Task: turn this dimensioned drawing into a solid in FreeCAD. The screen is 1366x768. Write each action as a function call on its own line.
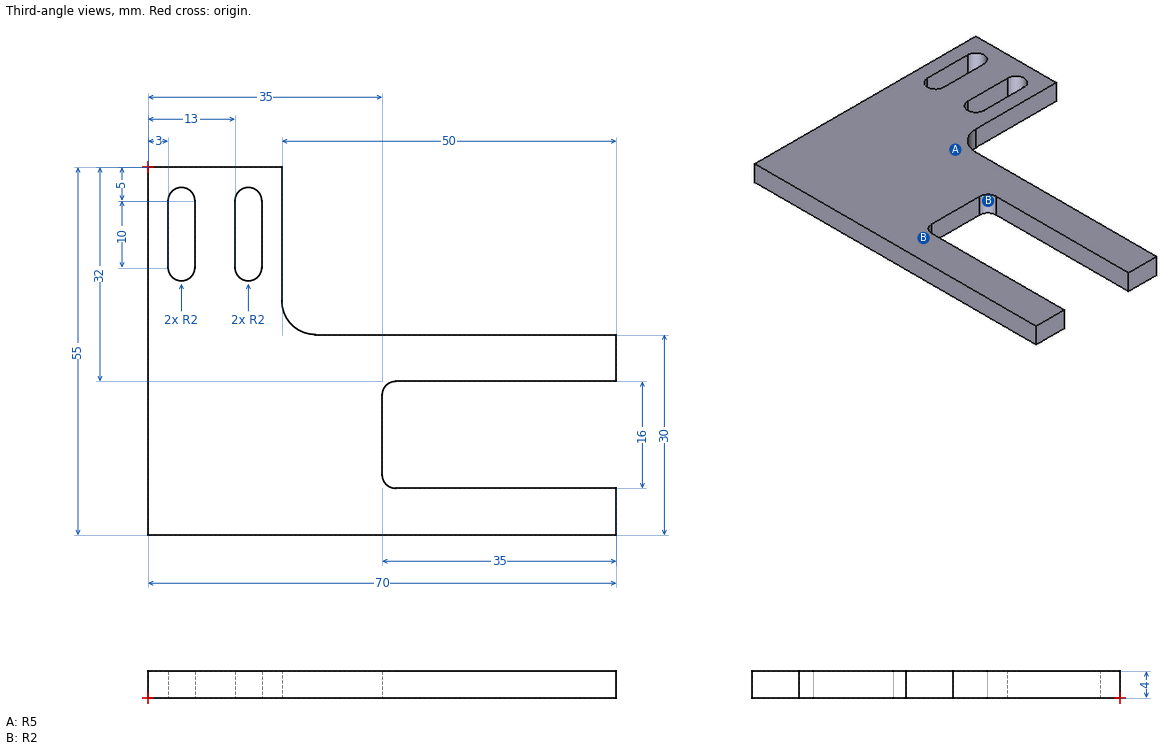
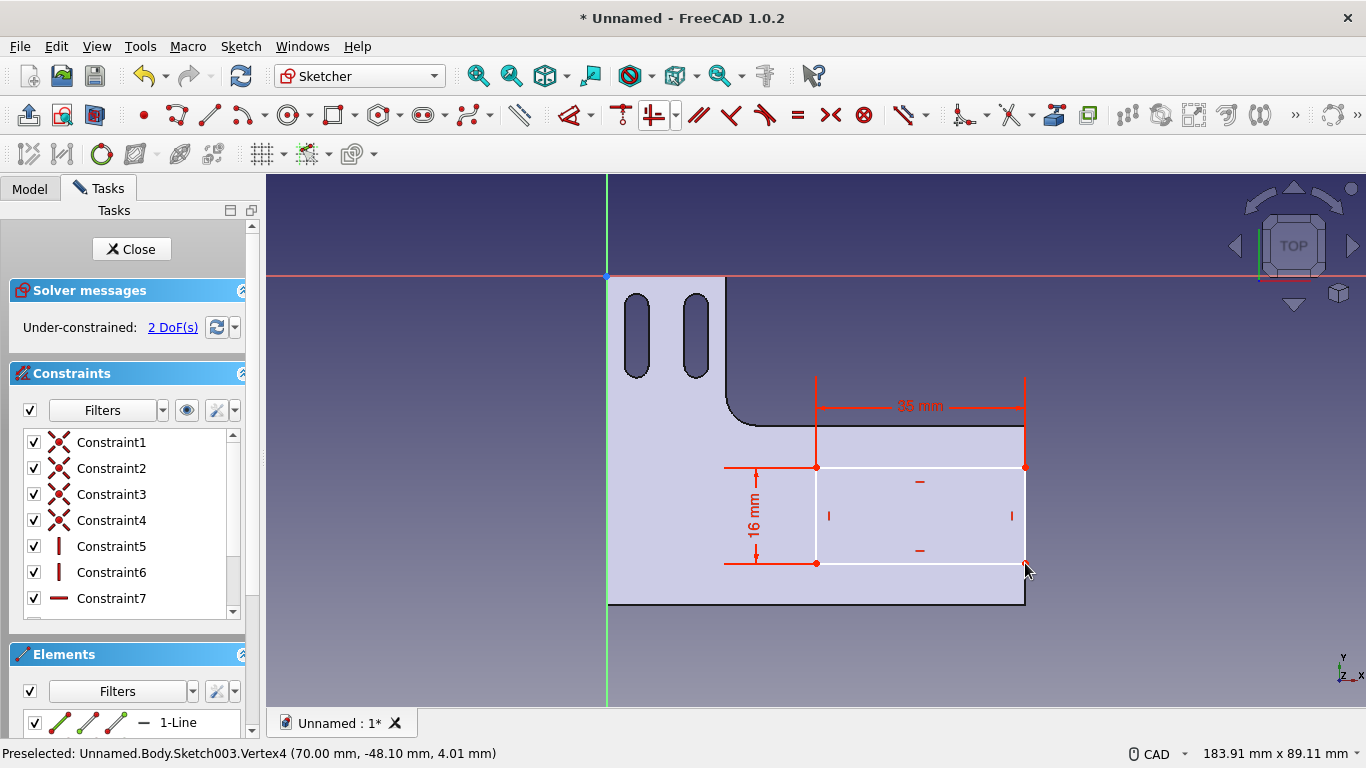
click(568, 116)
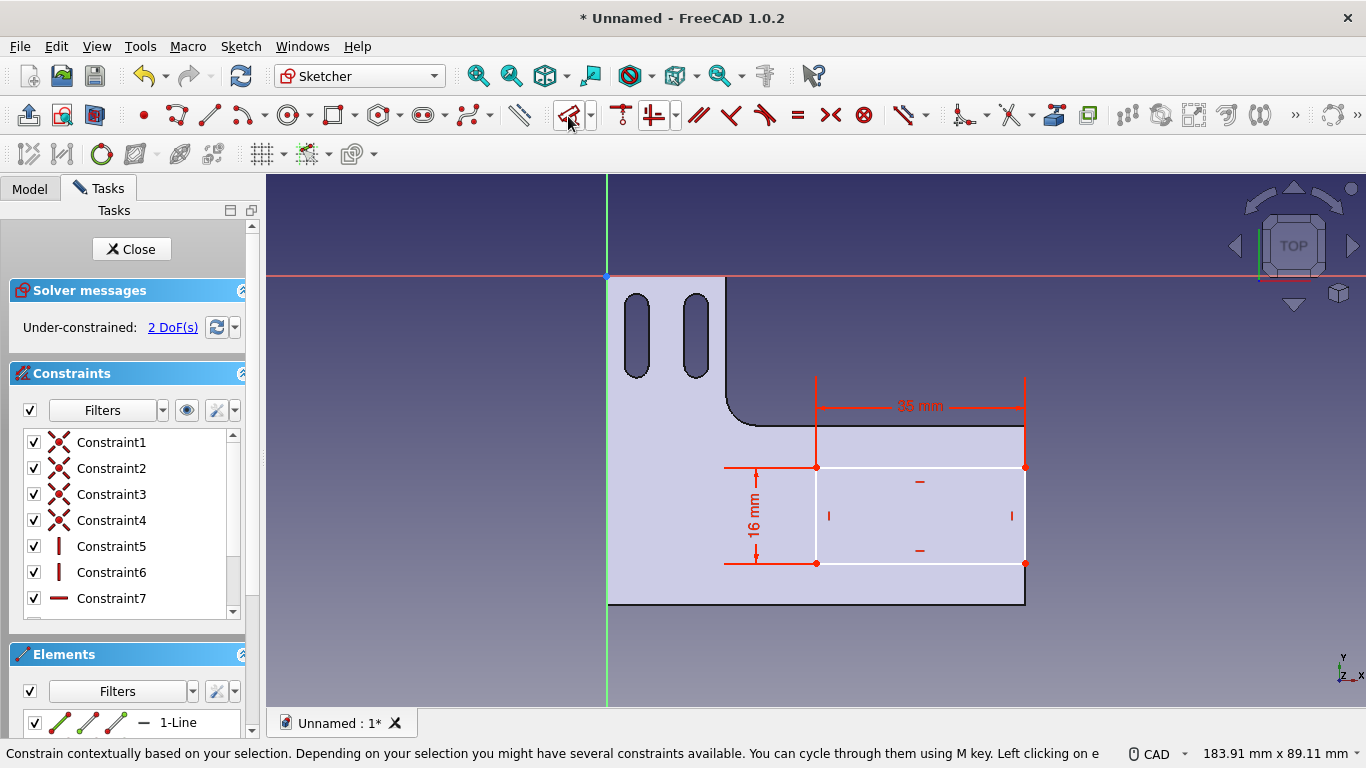
click(816, 468)
click(711, 242)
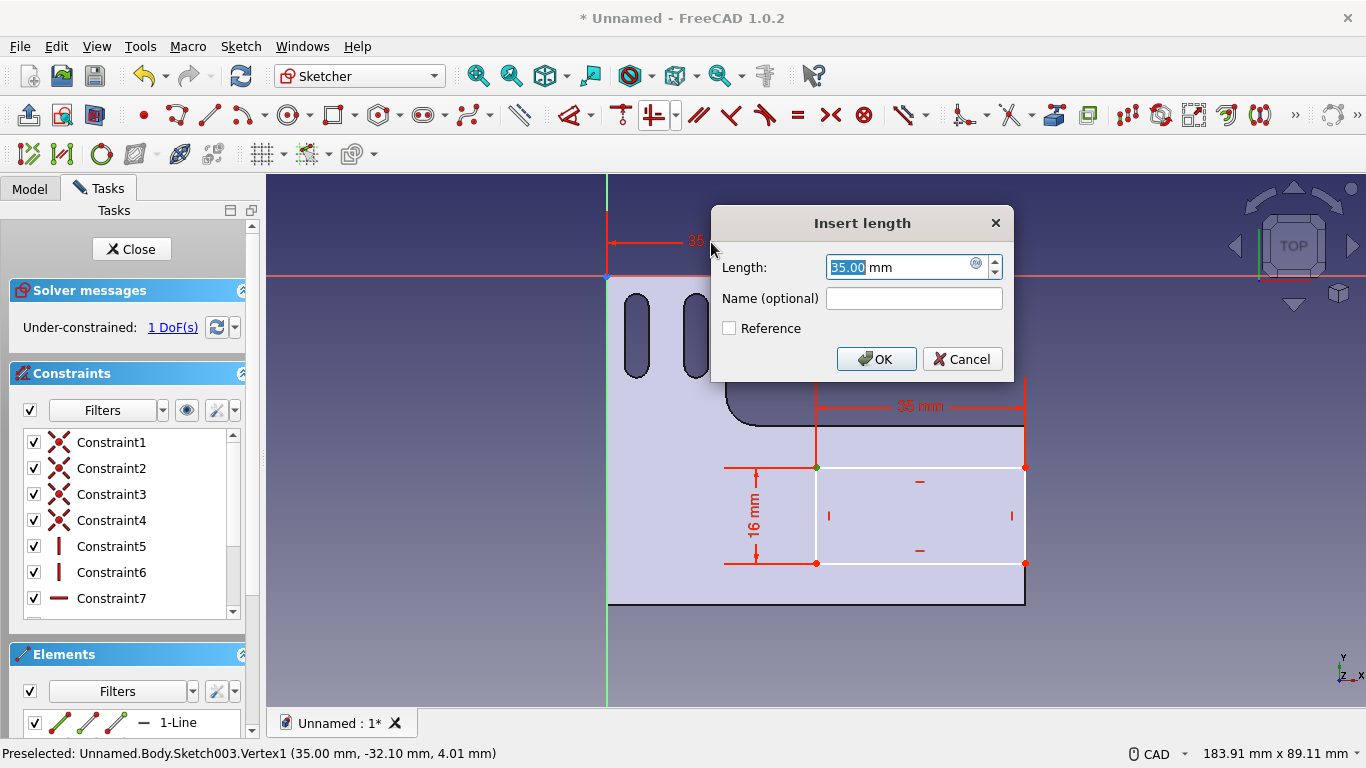
text(35)
key(Return)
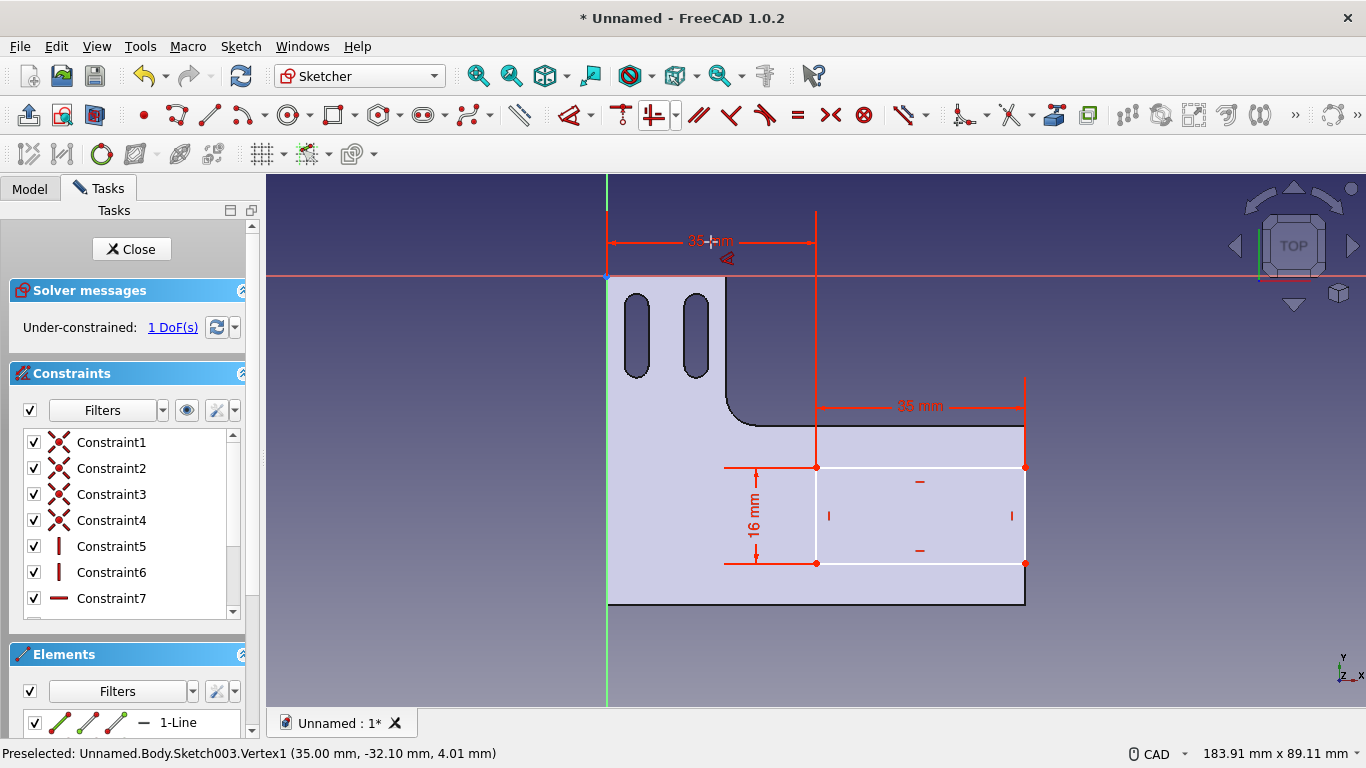
click(816, 468)
click(573, 372)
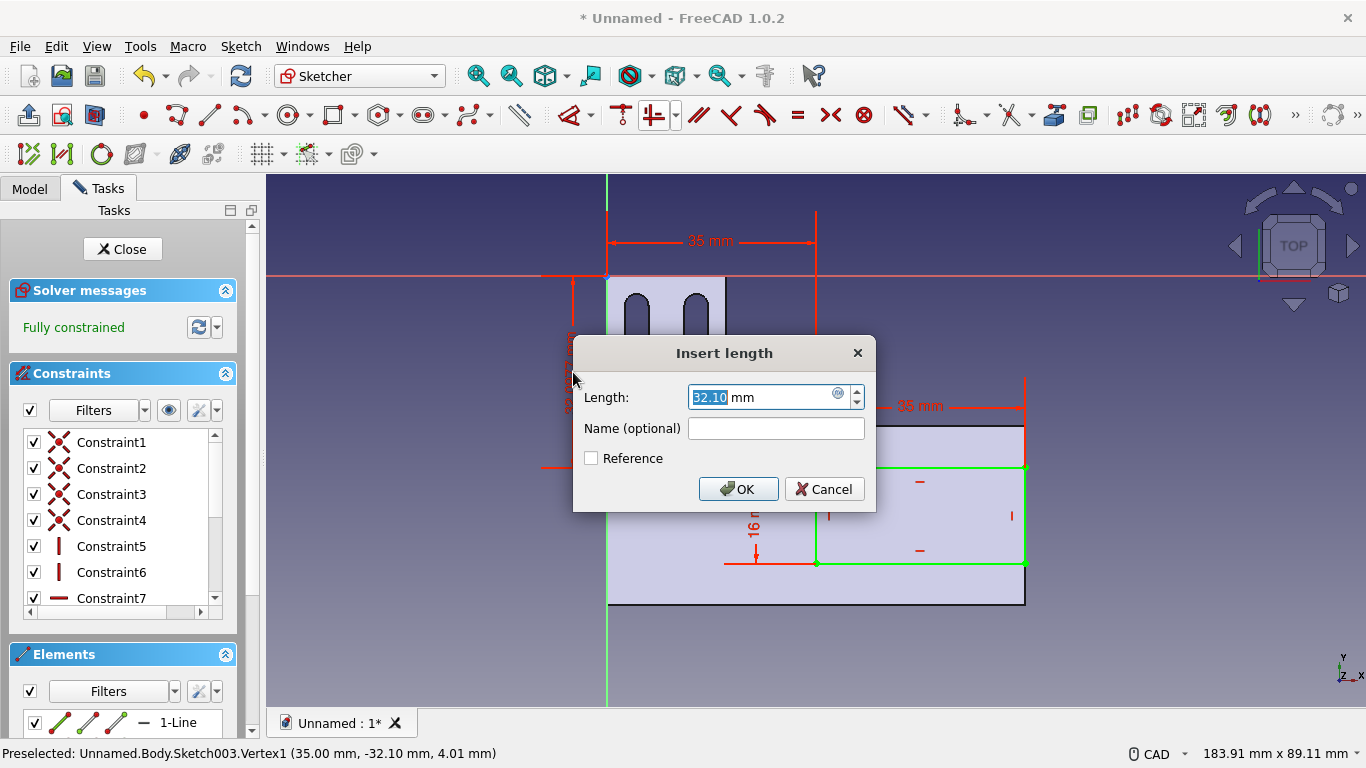
text(32)
key(Return)
key(Escape)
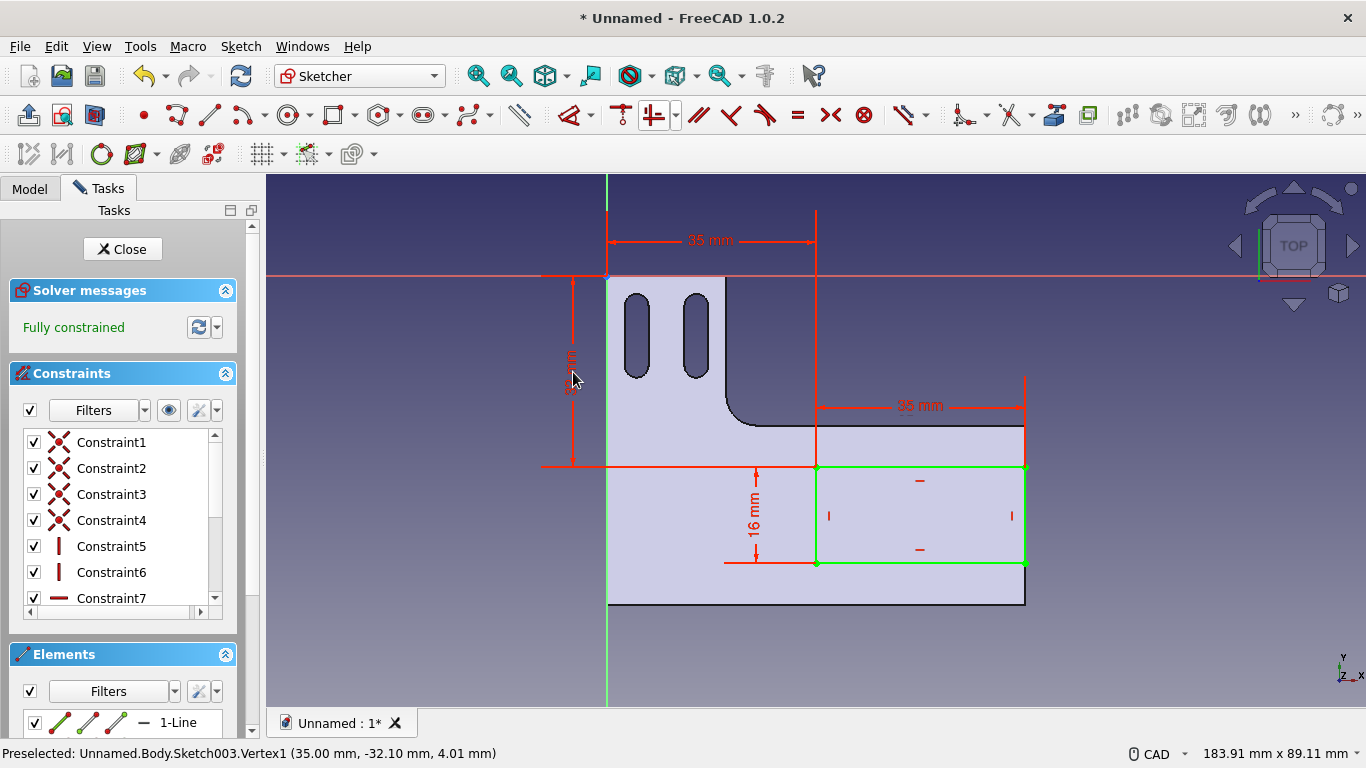
click(123, 249)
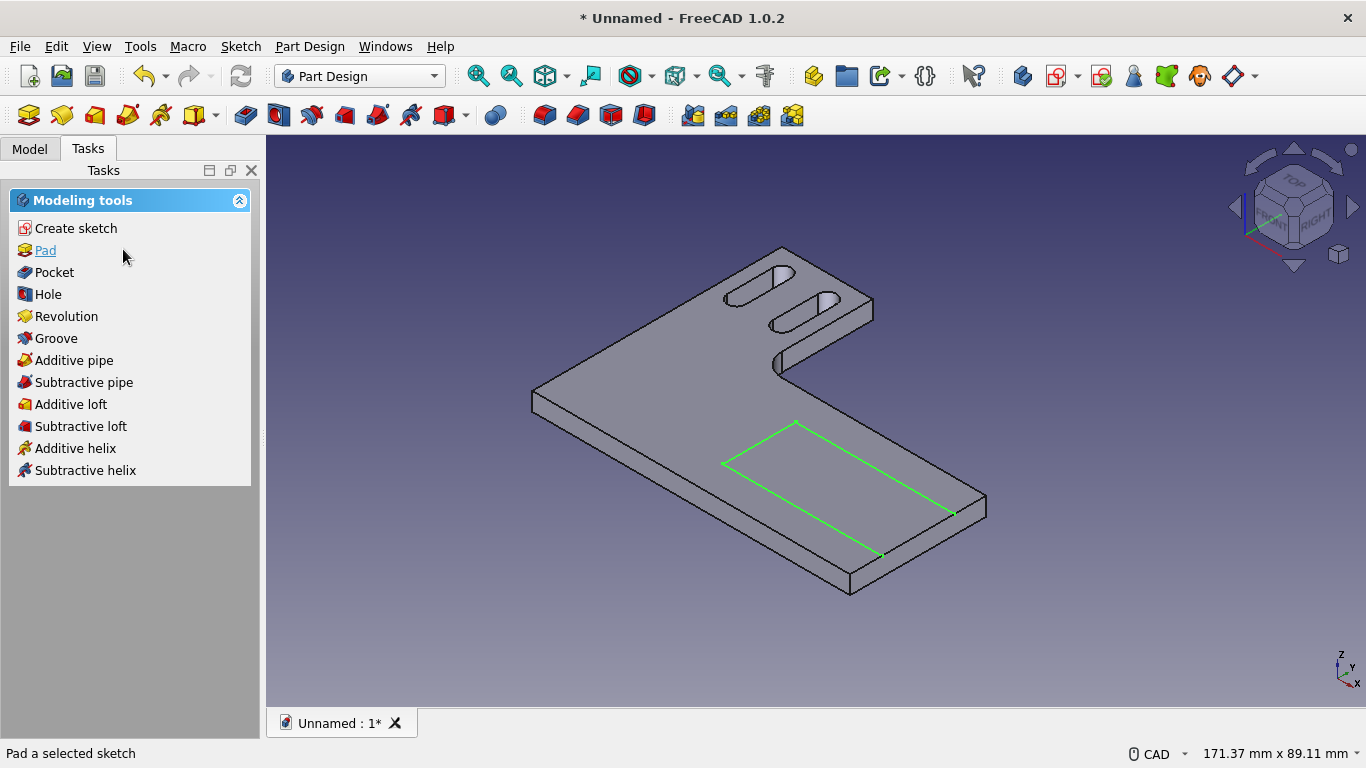
click(246, 116)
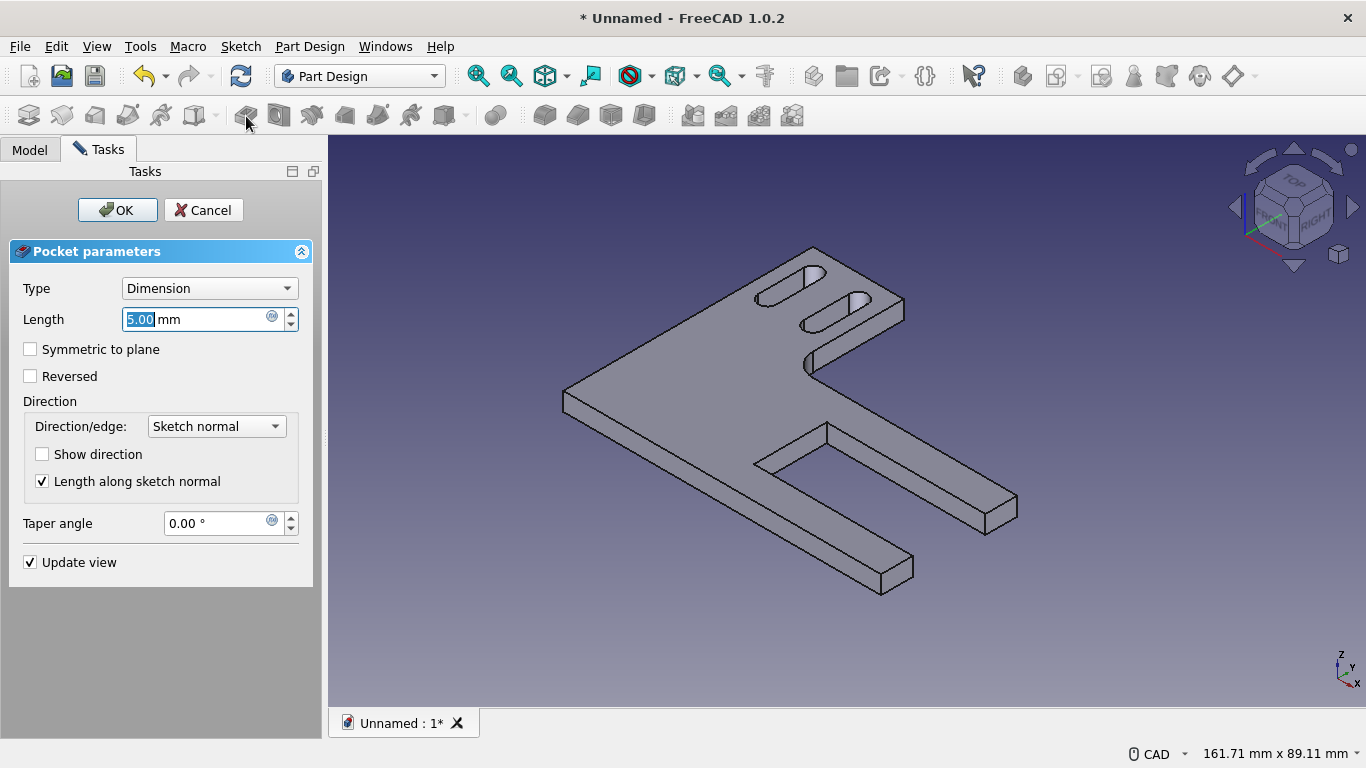
click(210, 288)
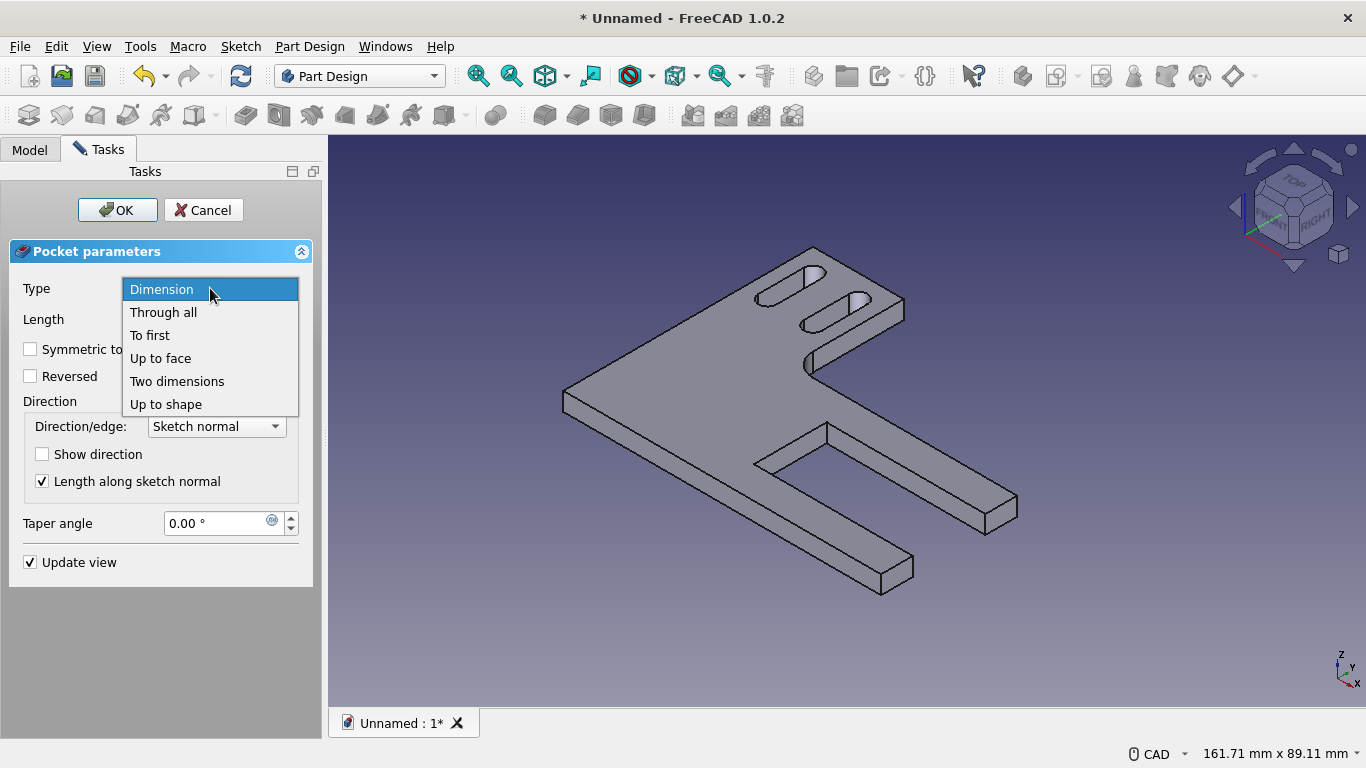
click(208, 336)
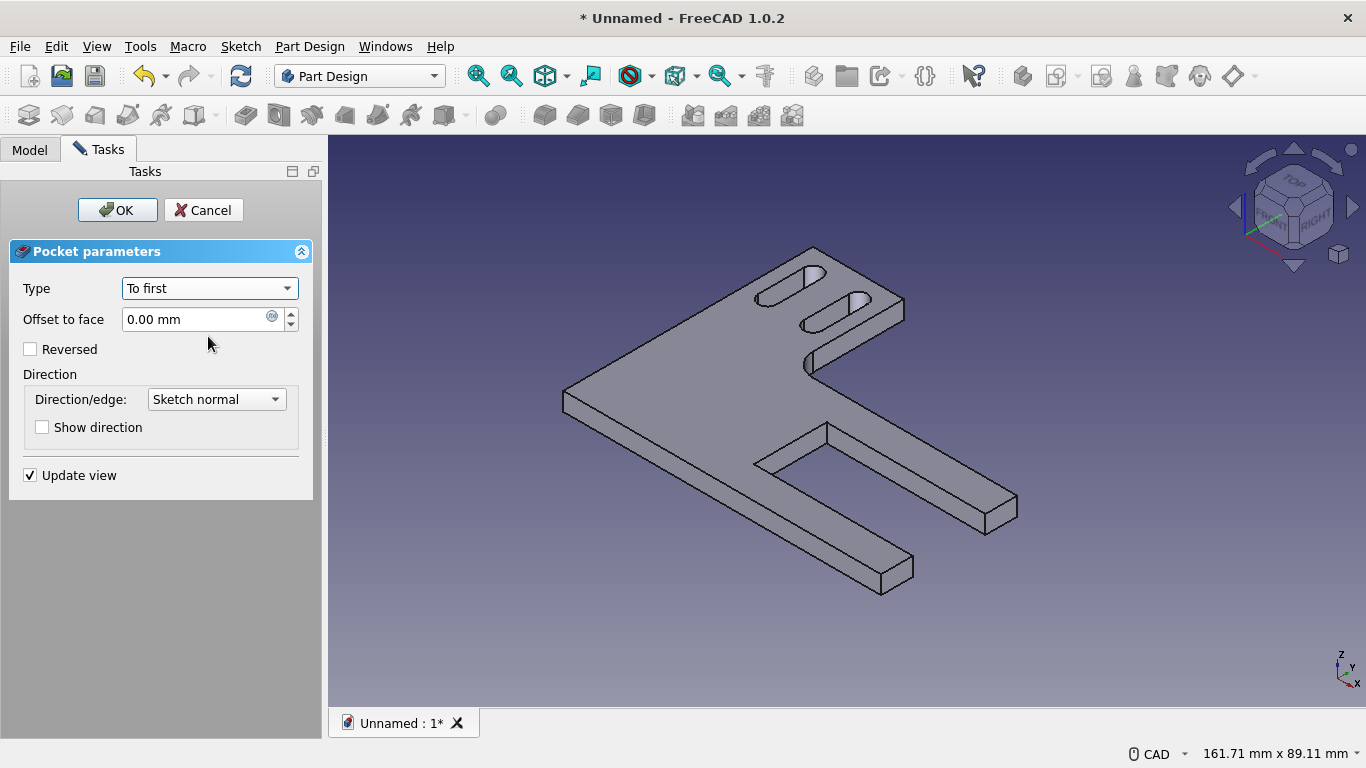
click(118, 210)